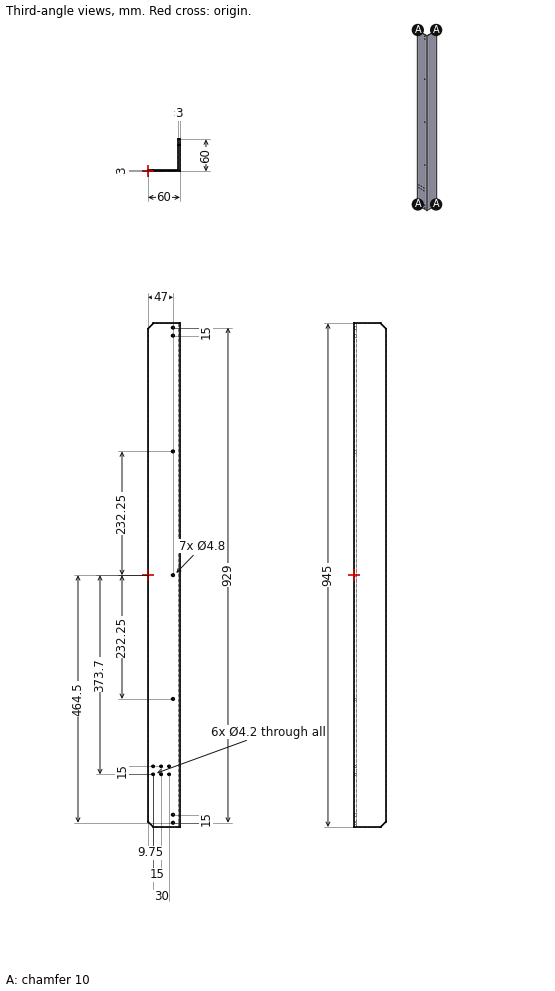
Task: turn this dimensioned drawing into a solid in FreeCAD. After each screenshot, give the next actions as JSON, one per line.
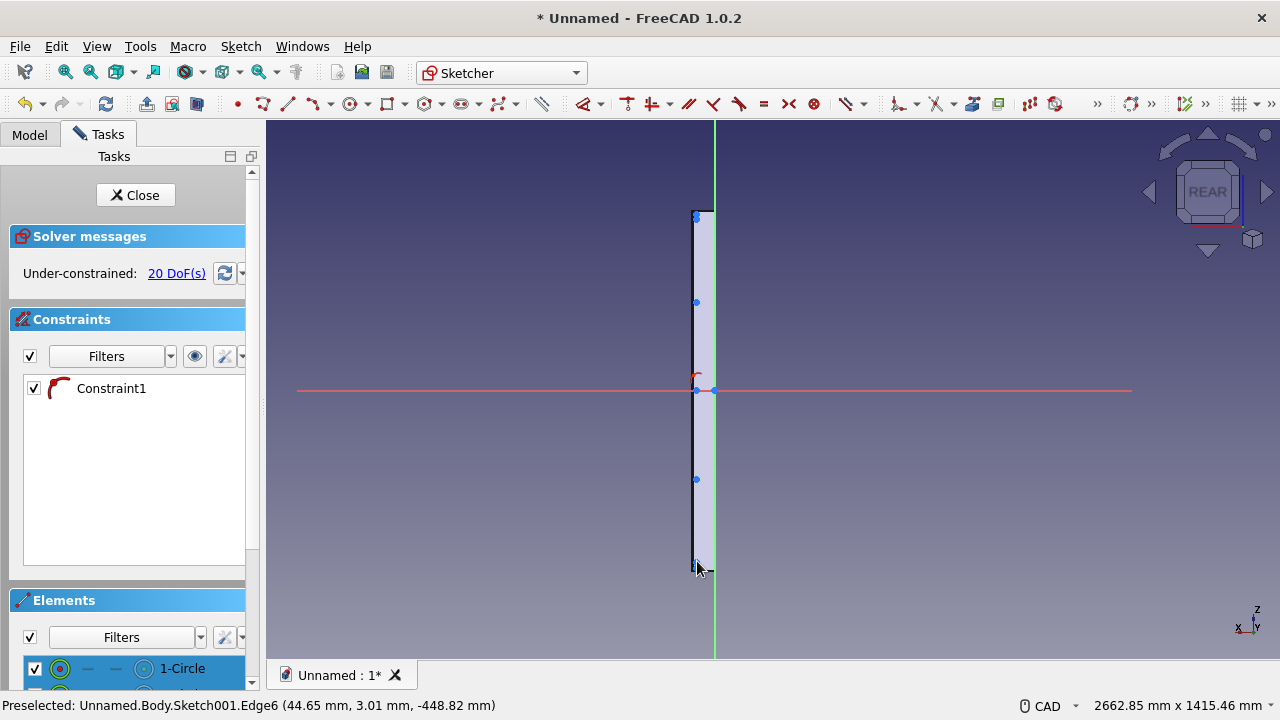
{"action": "scroll", "coordinate": [697, 219], "scroll_direction": "up", "scroll_amount": 14}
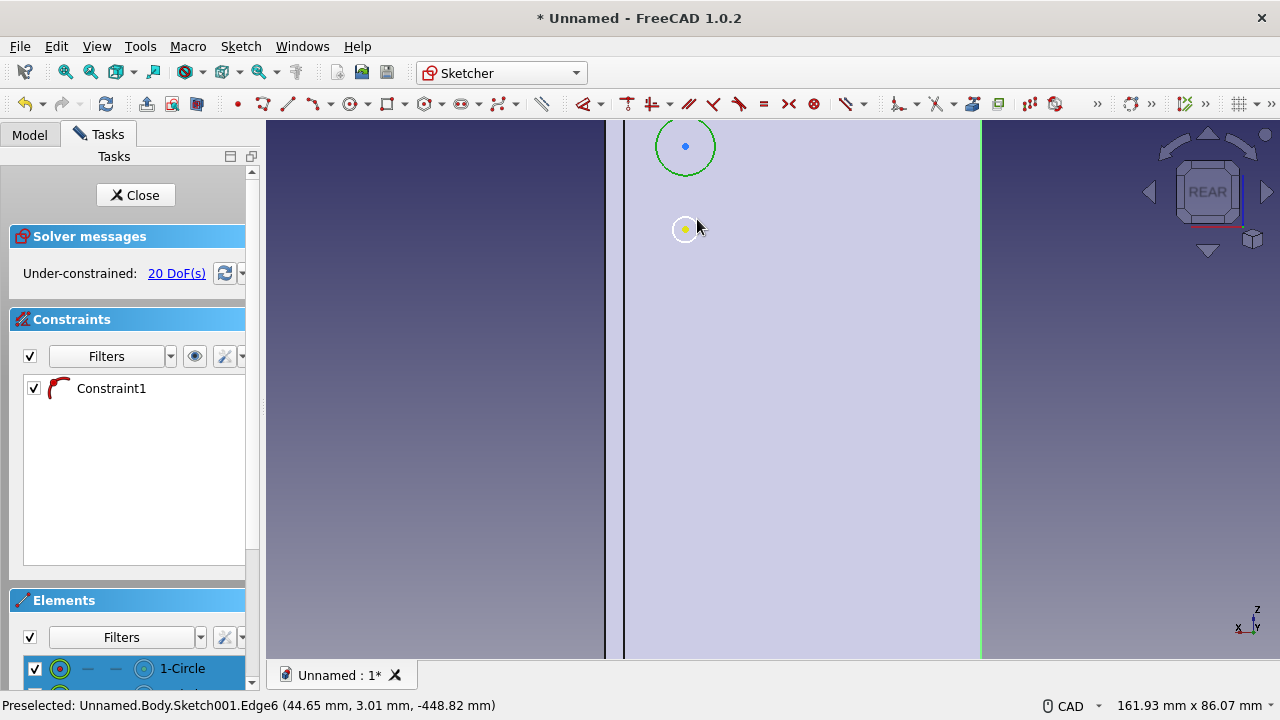
{"action": "left_click", "coordinate": [694, 221]}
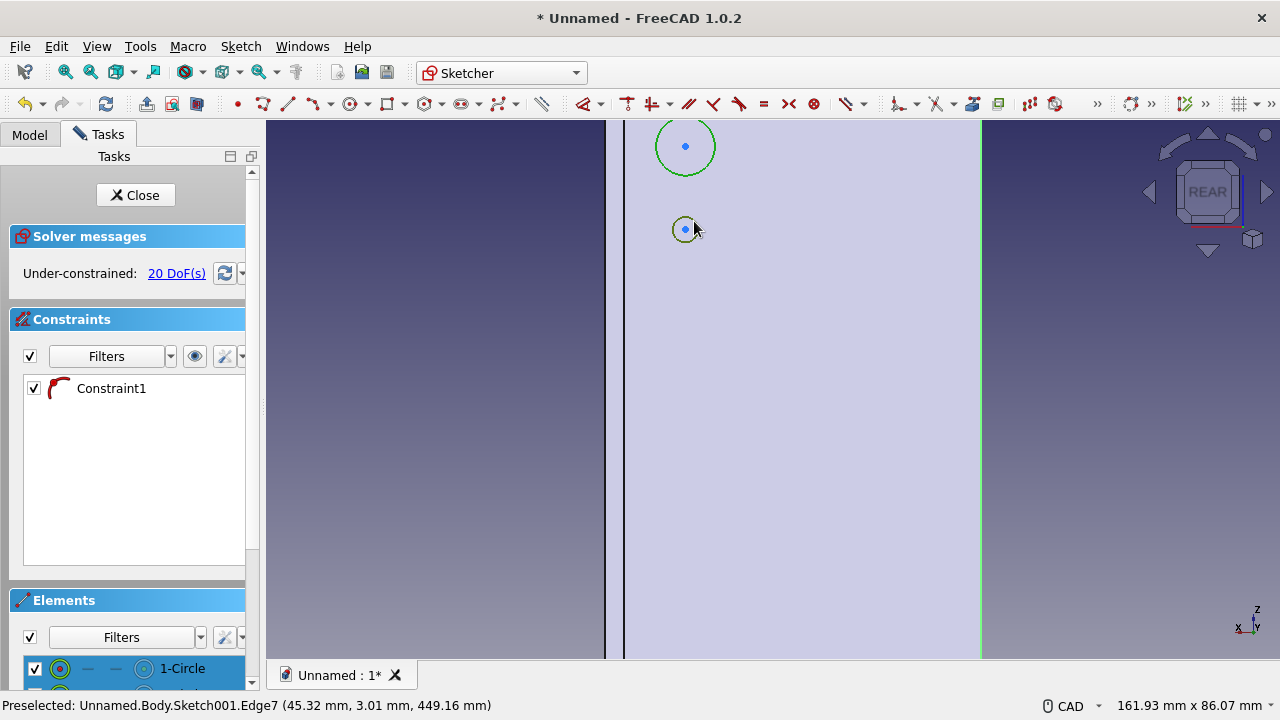
{"action": "left_click", "coordinate": [764, 104]}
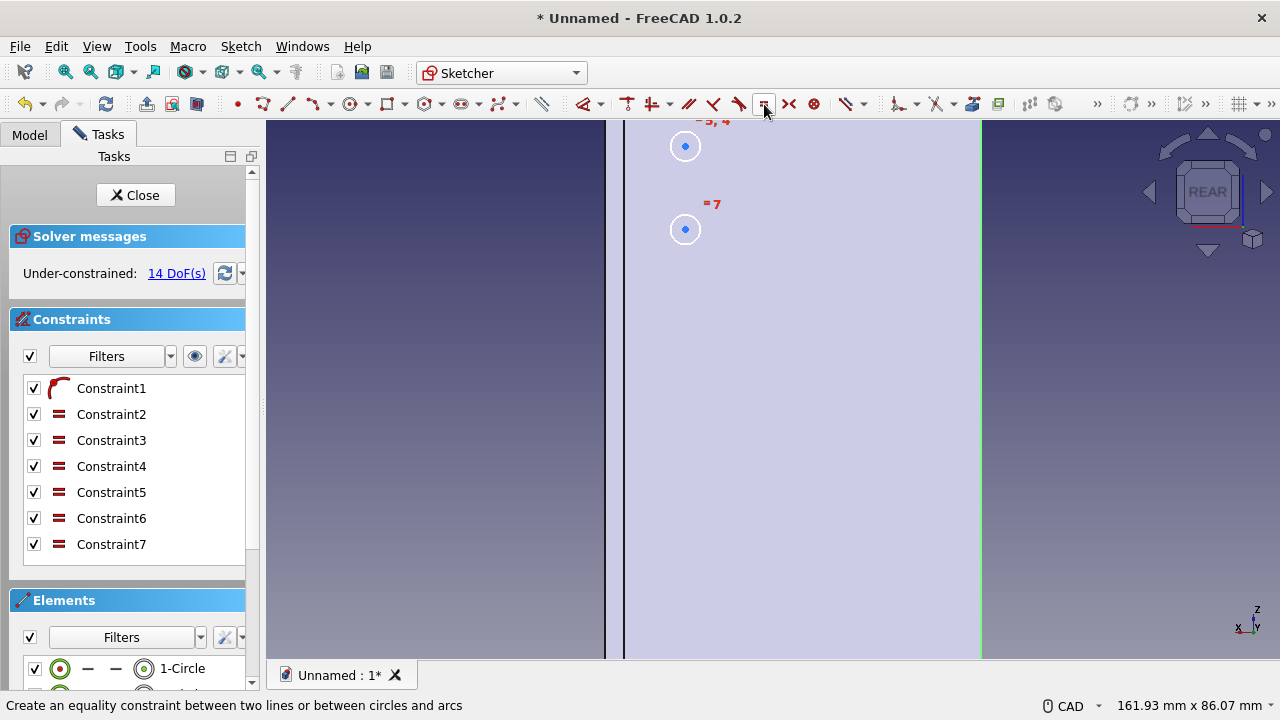
{"action": "scroll", "coordinate": [697, 218], "scroll_direction": "down", "scroll_amount": 14}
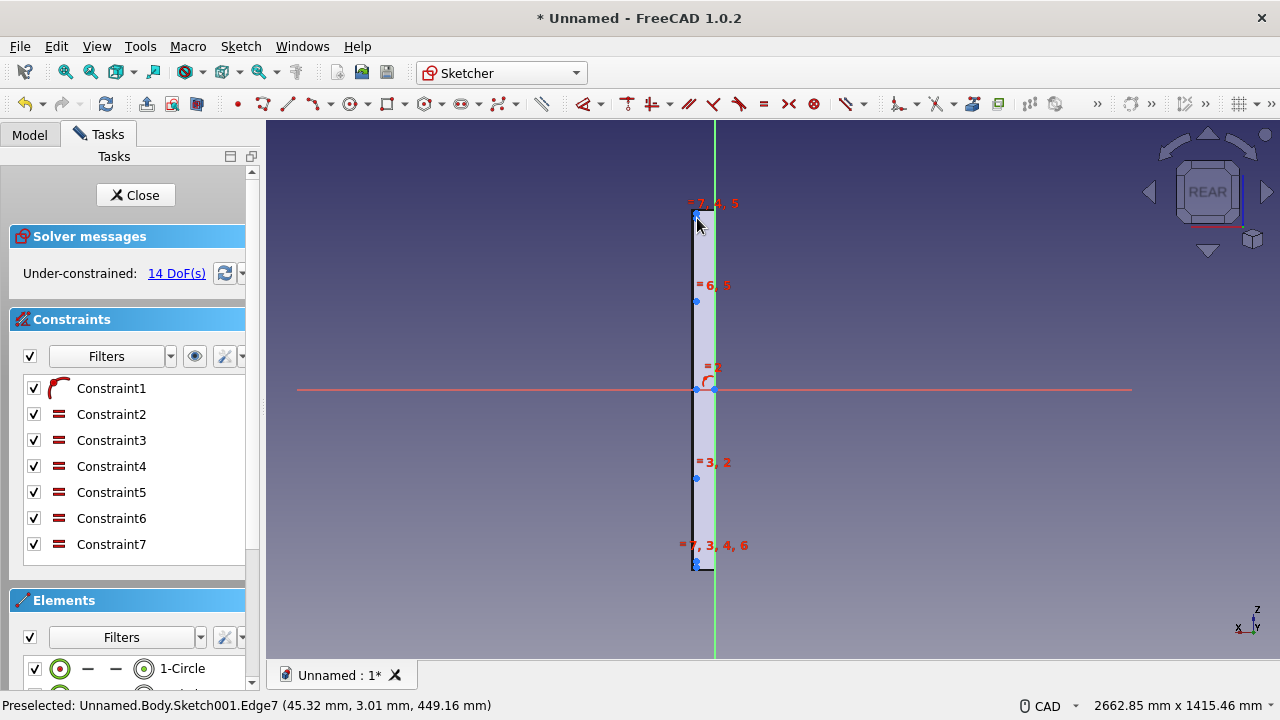
{"action": "left_click", "coordinate": [697, 390]}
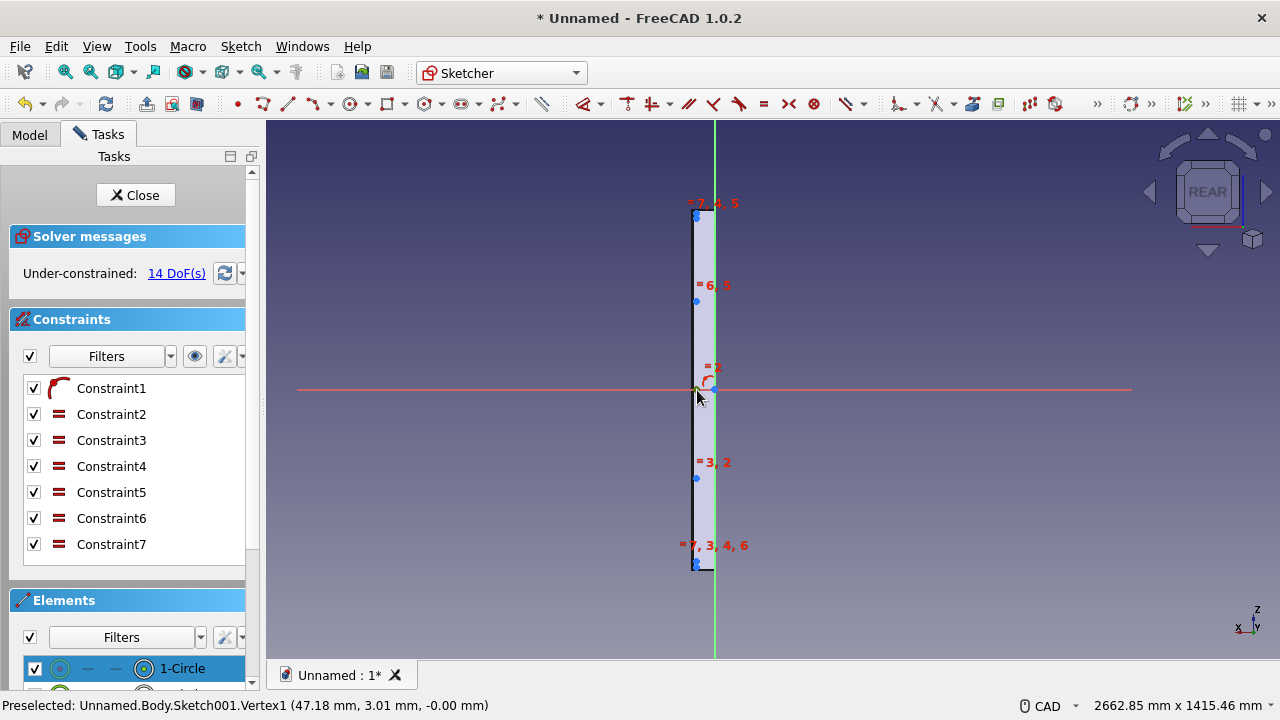
{"action": "left_click", "coordinate": [697, 479]}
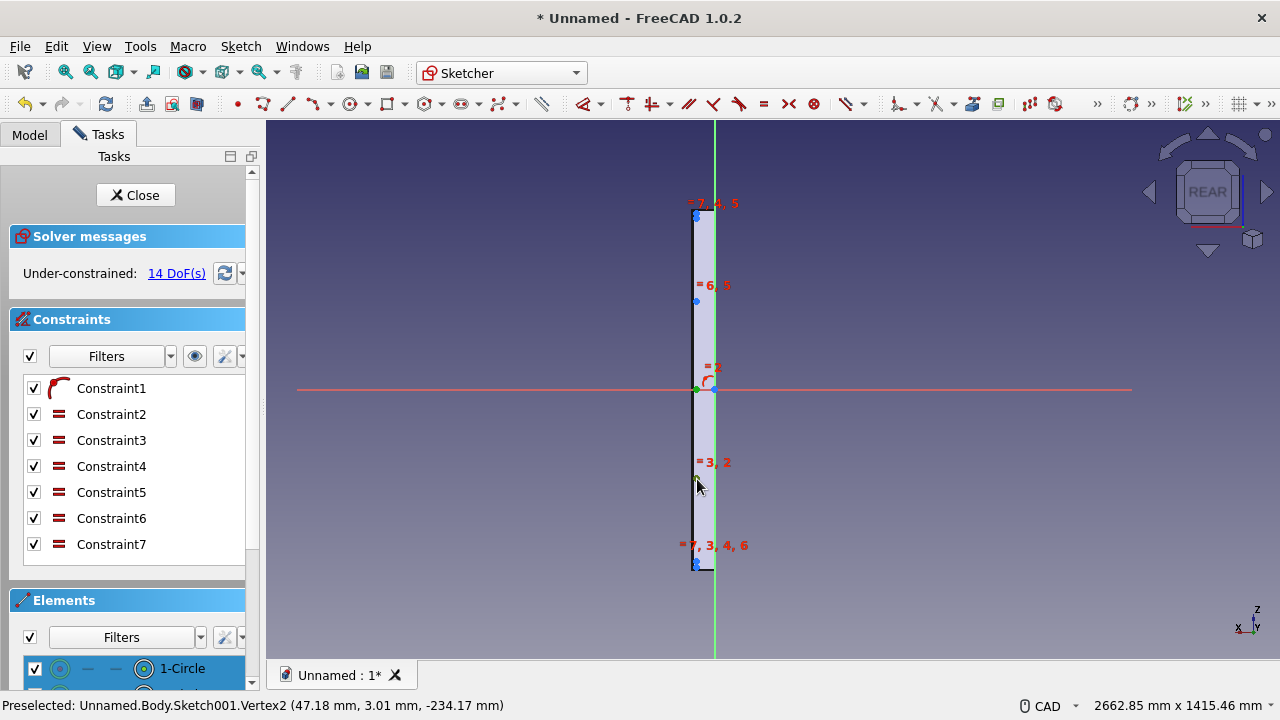
{"action": "left_click", "coordinate": [670, 104]}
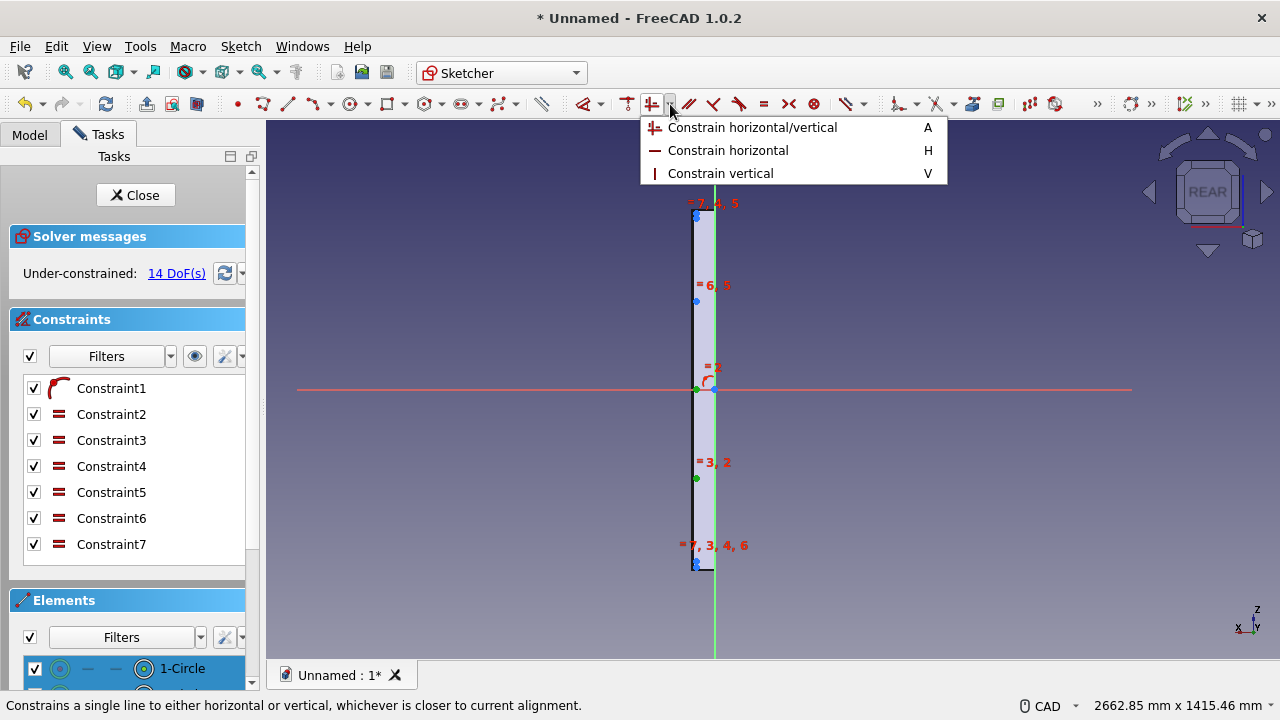
{"action": "left_click", "coordinate": [794, 174]}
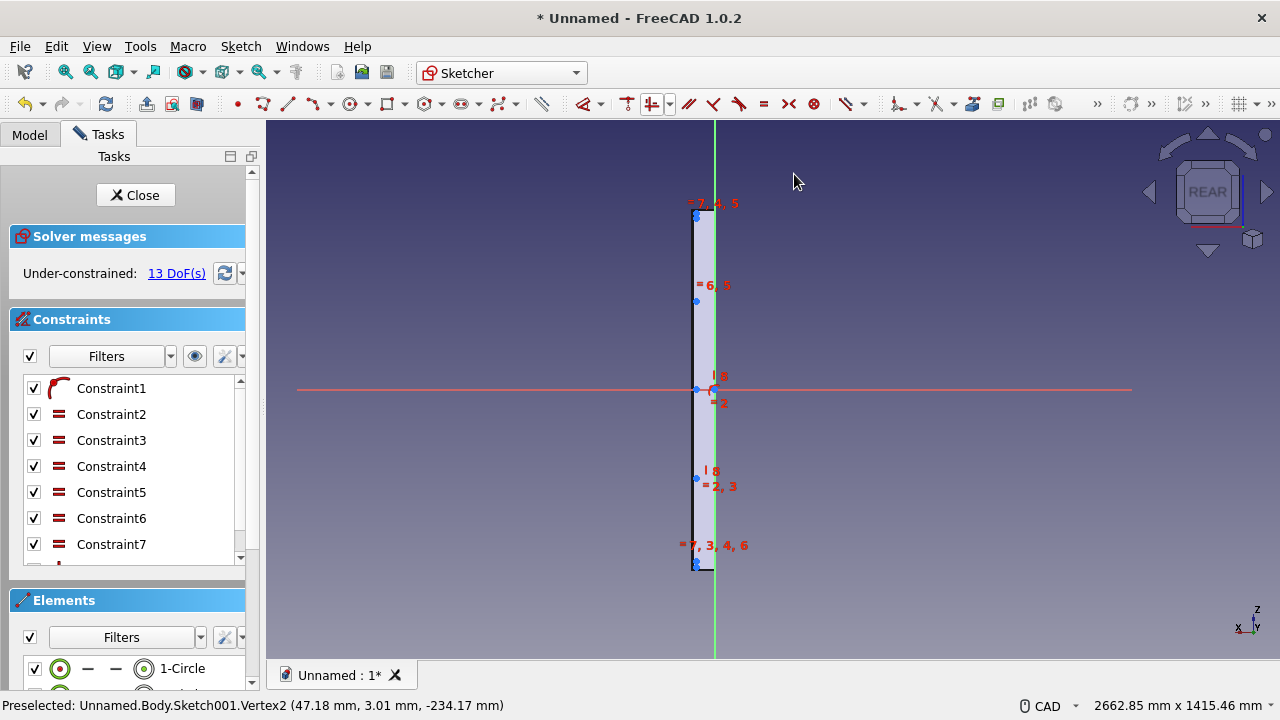
{"action": "left_click", "coordinate": [697, 479]}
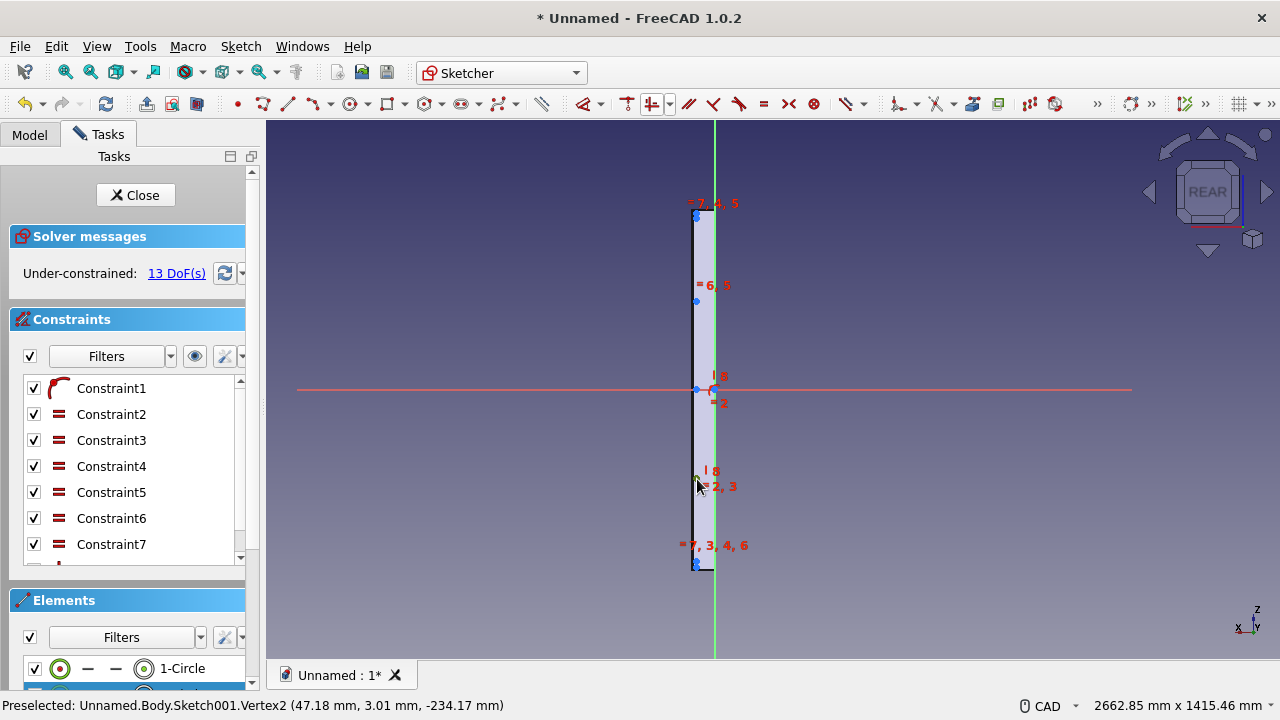
{"action": "scroll", "coordinate": [697, 568], "scroll_direction": "up", "scroll_amount": 3}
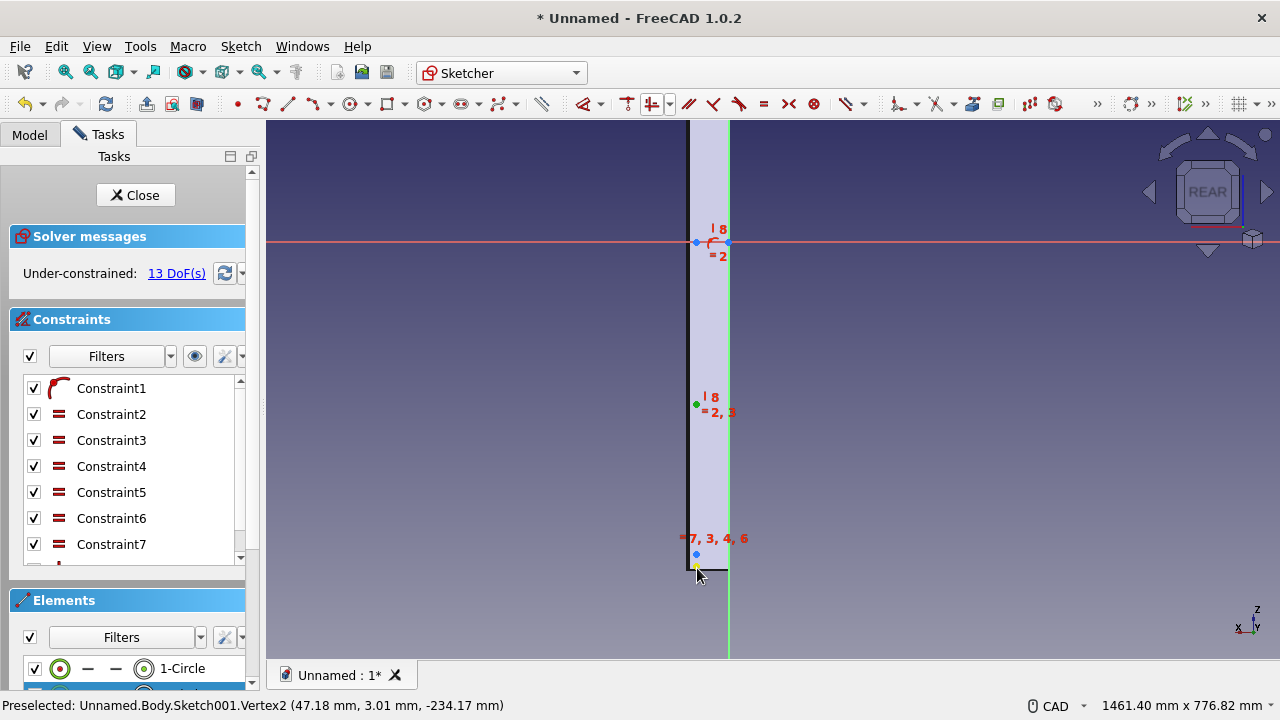
{"action": "left_click", "coordinate": [696, 567]}